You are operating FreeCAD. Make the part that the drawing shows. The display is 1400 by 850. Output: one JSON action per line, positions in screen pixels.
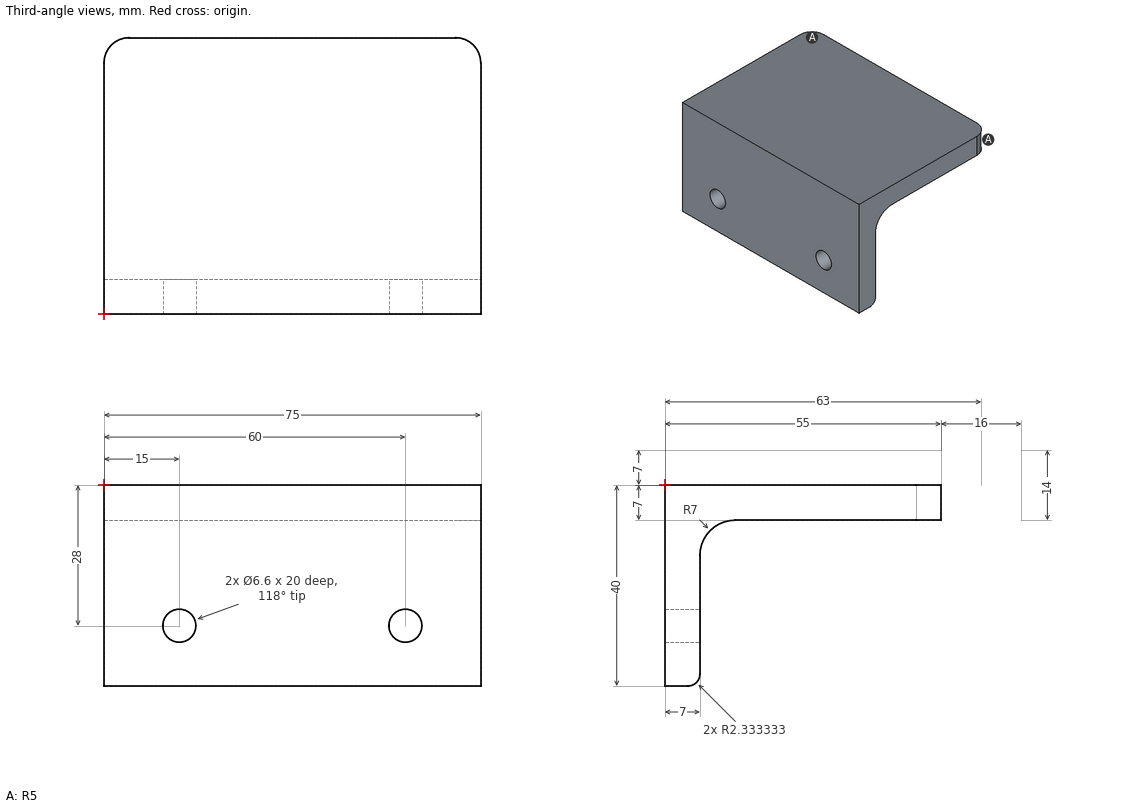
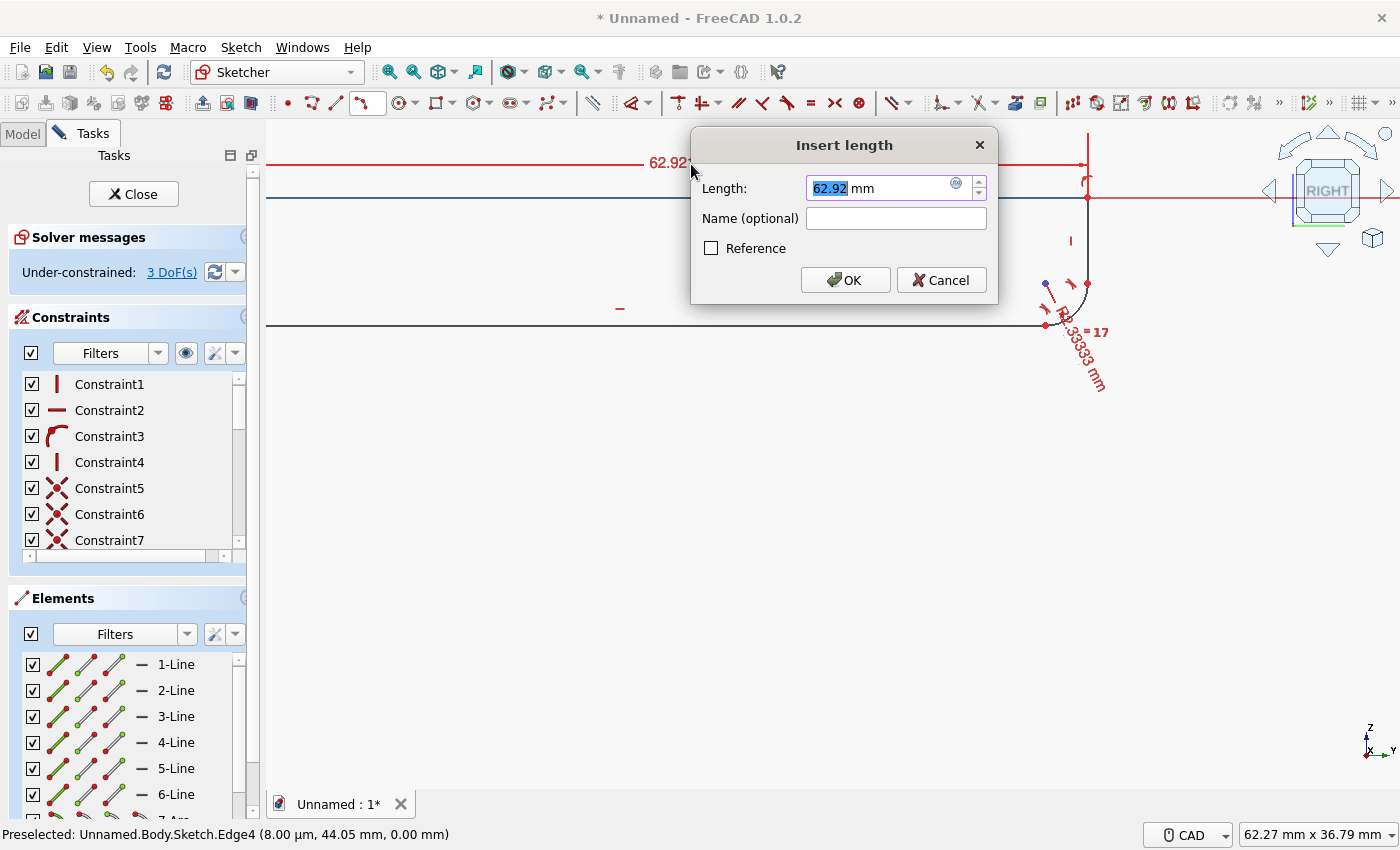
{"action": "type", "text": "63"}
{"action": "key", "text": "Return"}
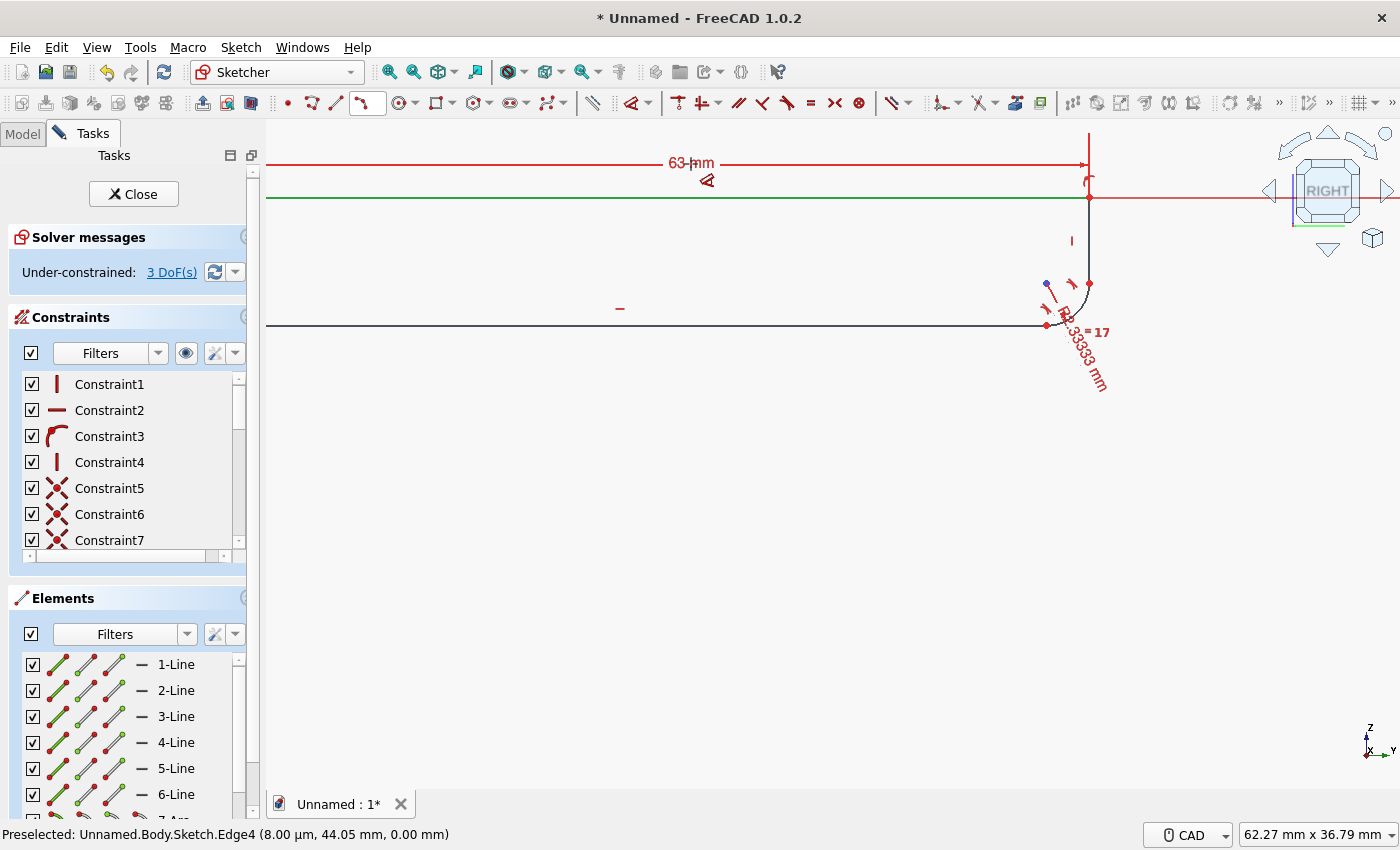
{"action": "scroll", "coordinate": [1067, 323], "scroll_direction": "down", "scroll_amount": 3}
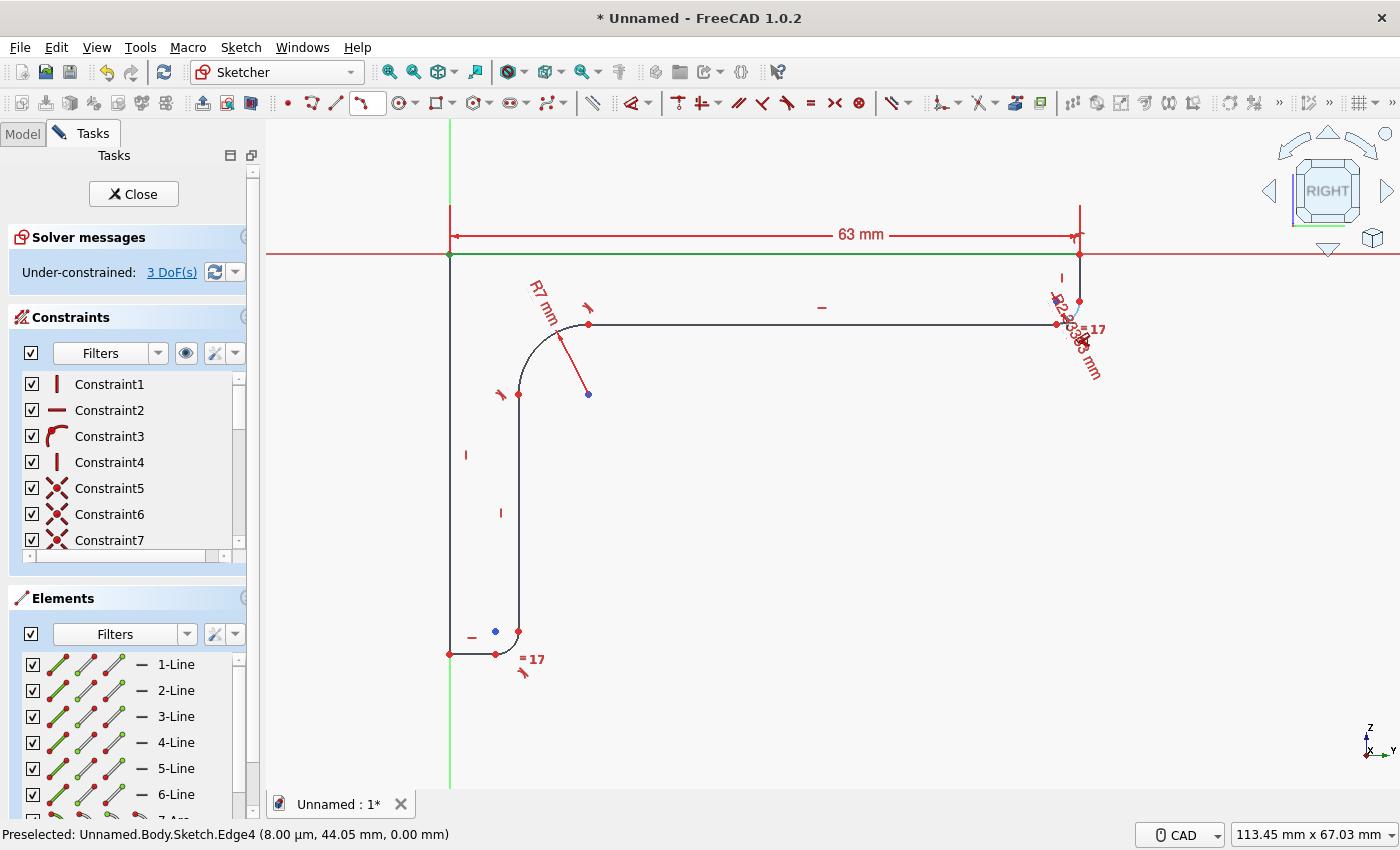
{"action": "left_click", "coordinate": [450, 374]}
{"action": "left_click", "coordinate": [416, 454]}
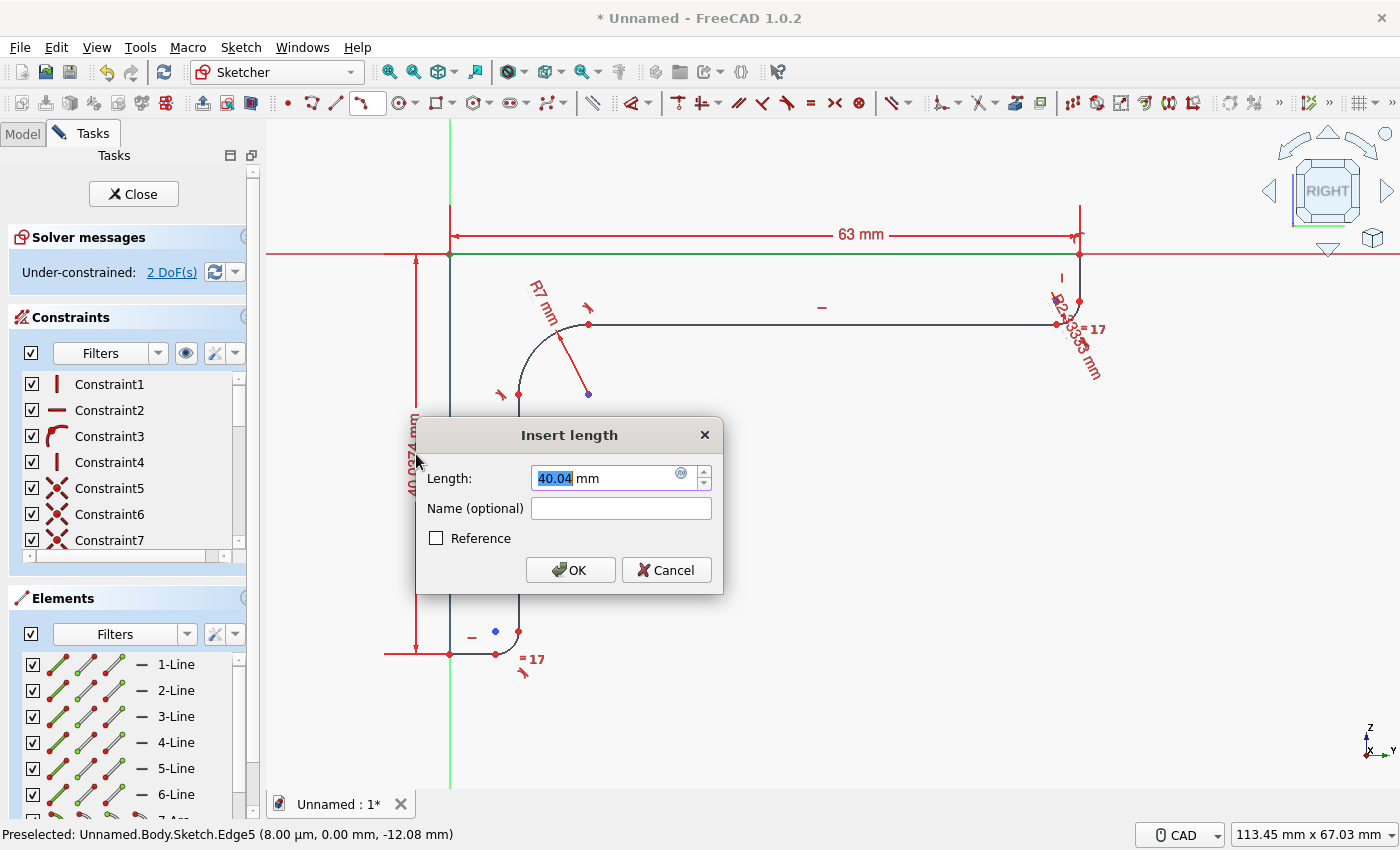
{"action": "type", "text": "40"}
{"action": "key", "text": "Return"}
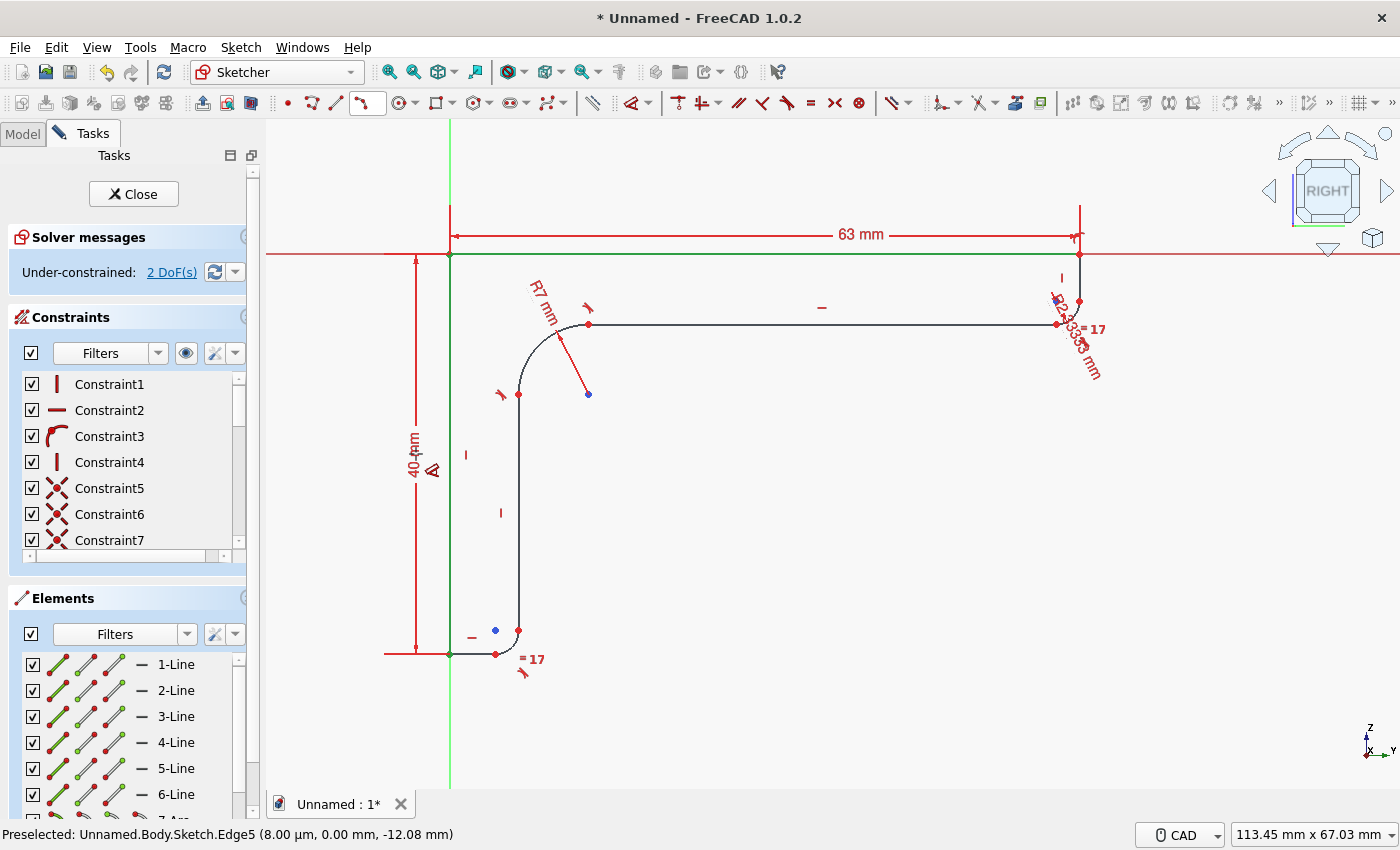
{"action": "left_click", "coordinate": [519, 631]}
{"action": "left_click", "coordinate": [484, 220]}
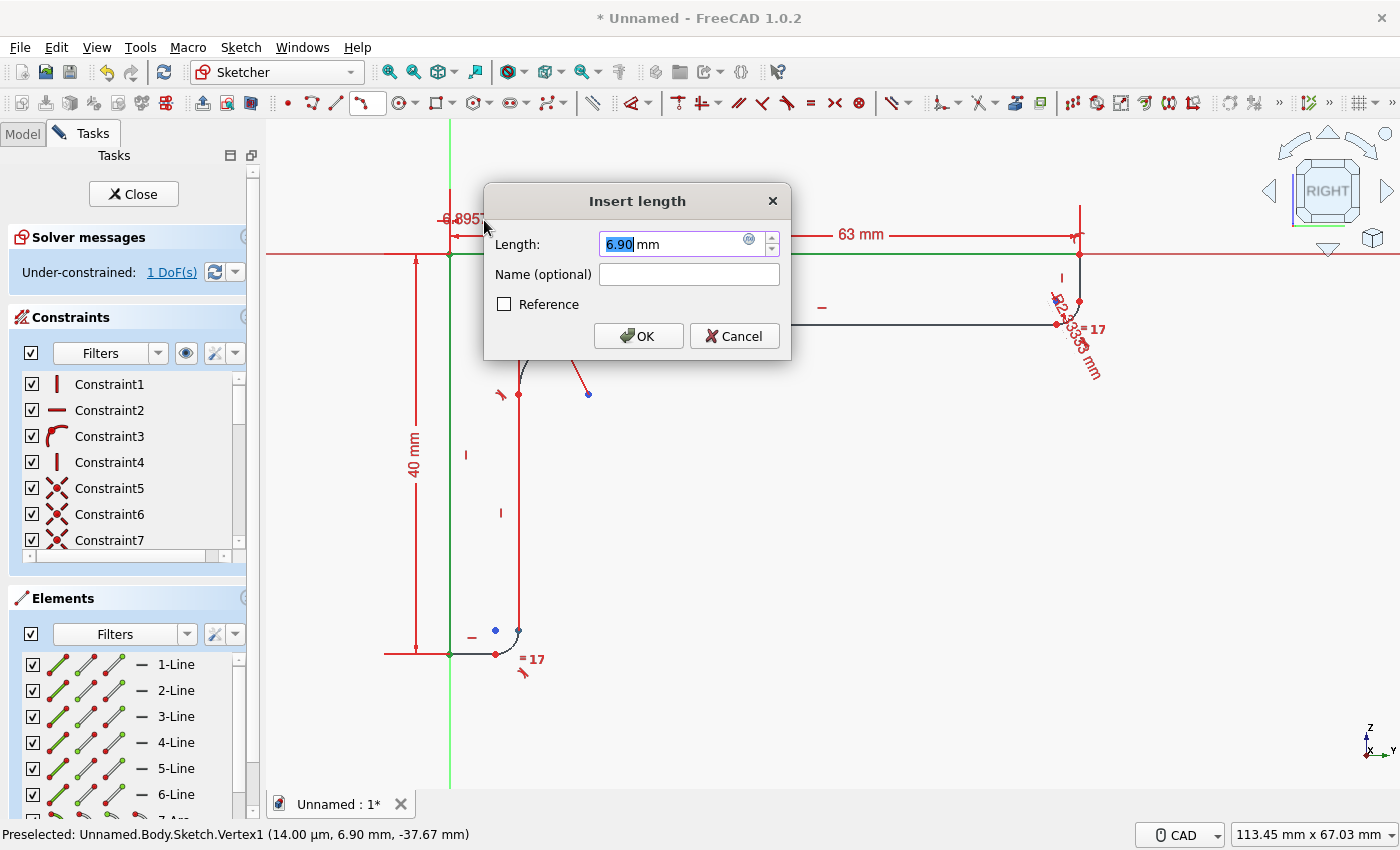
{"action": "type", "text": "7"}
{"action": "key", "text": "Return"}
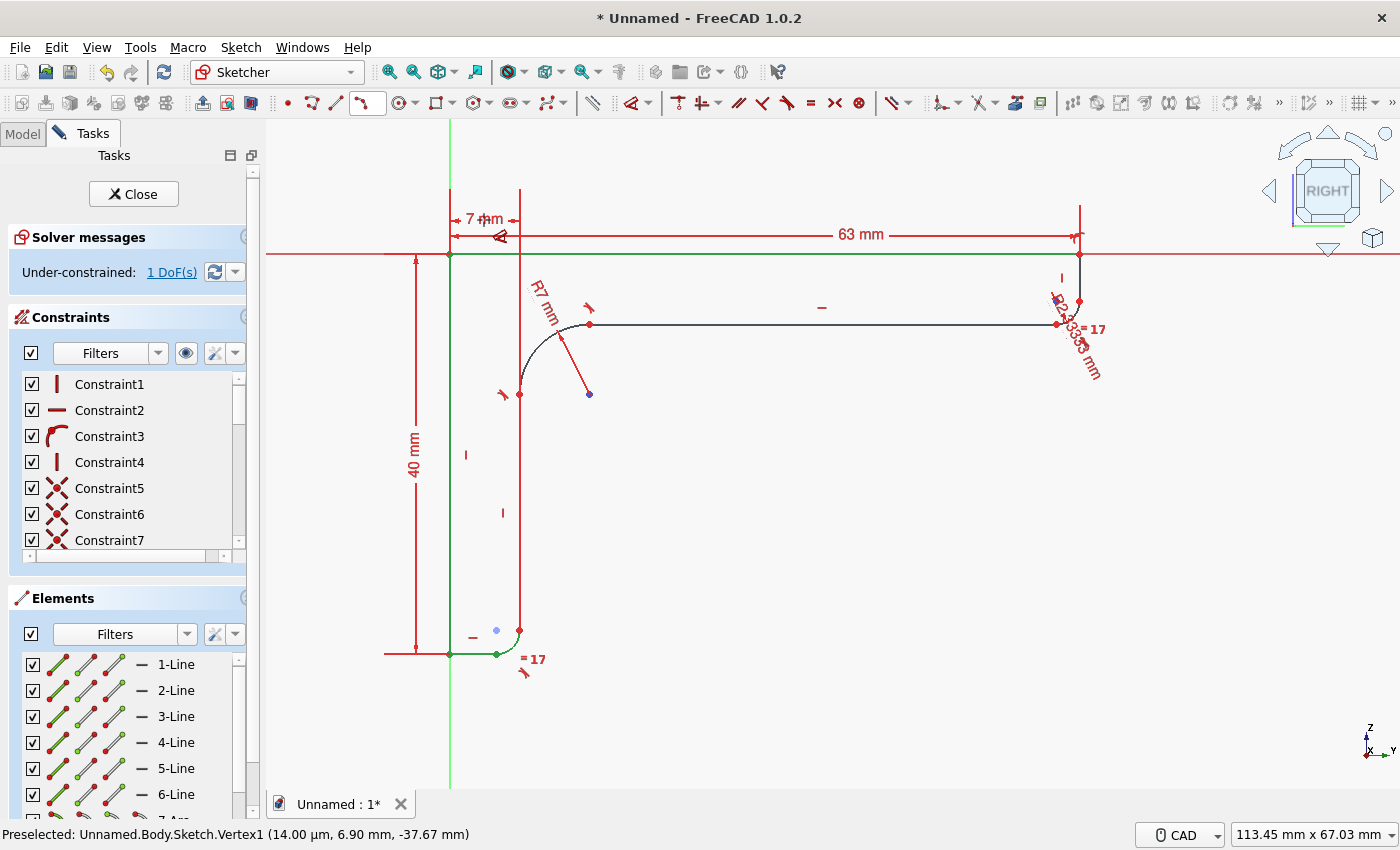
{"action": "left_click", "coordinate": [590, 325]}
{"action": "left_click", "coordinate": [416, 289]}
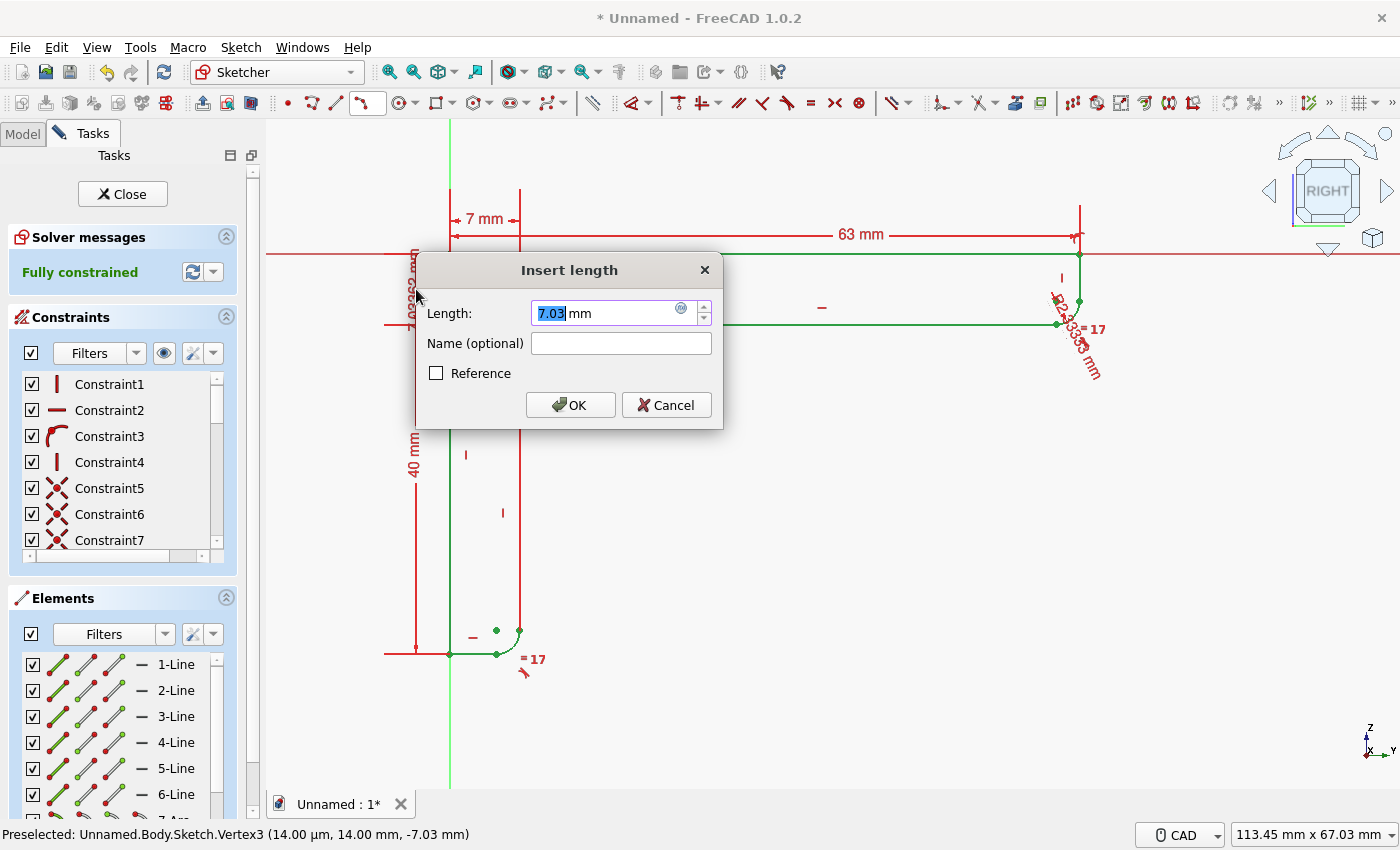
{"action": "type", "text": "7"}
{"action": "key", "text": "Return"}
{"action": "key", "text": "Escape"}